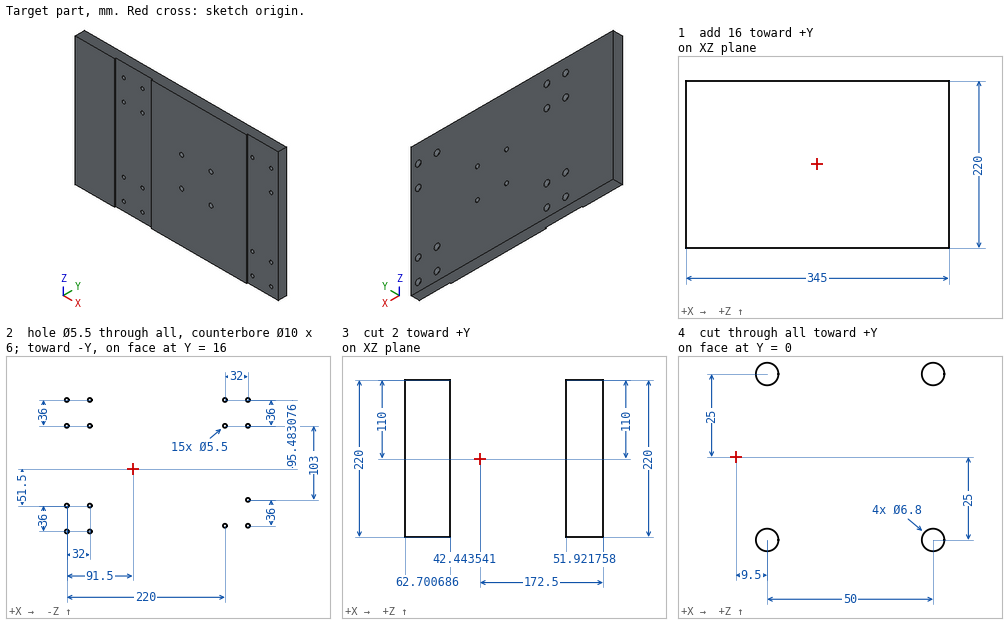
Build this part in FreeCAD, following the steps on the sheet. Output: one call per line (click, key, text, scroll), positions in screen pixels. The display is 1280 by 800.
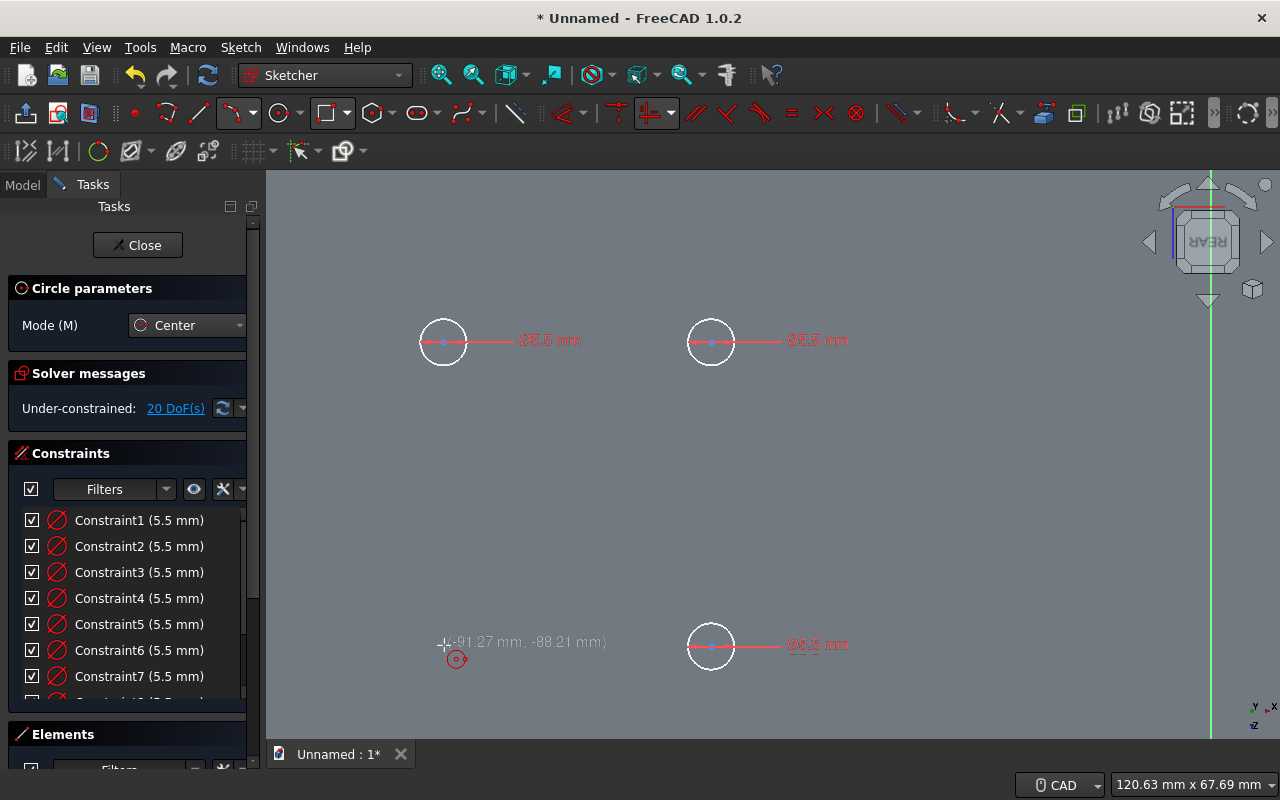
scroll(444, 645, down, 7)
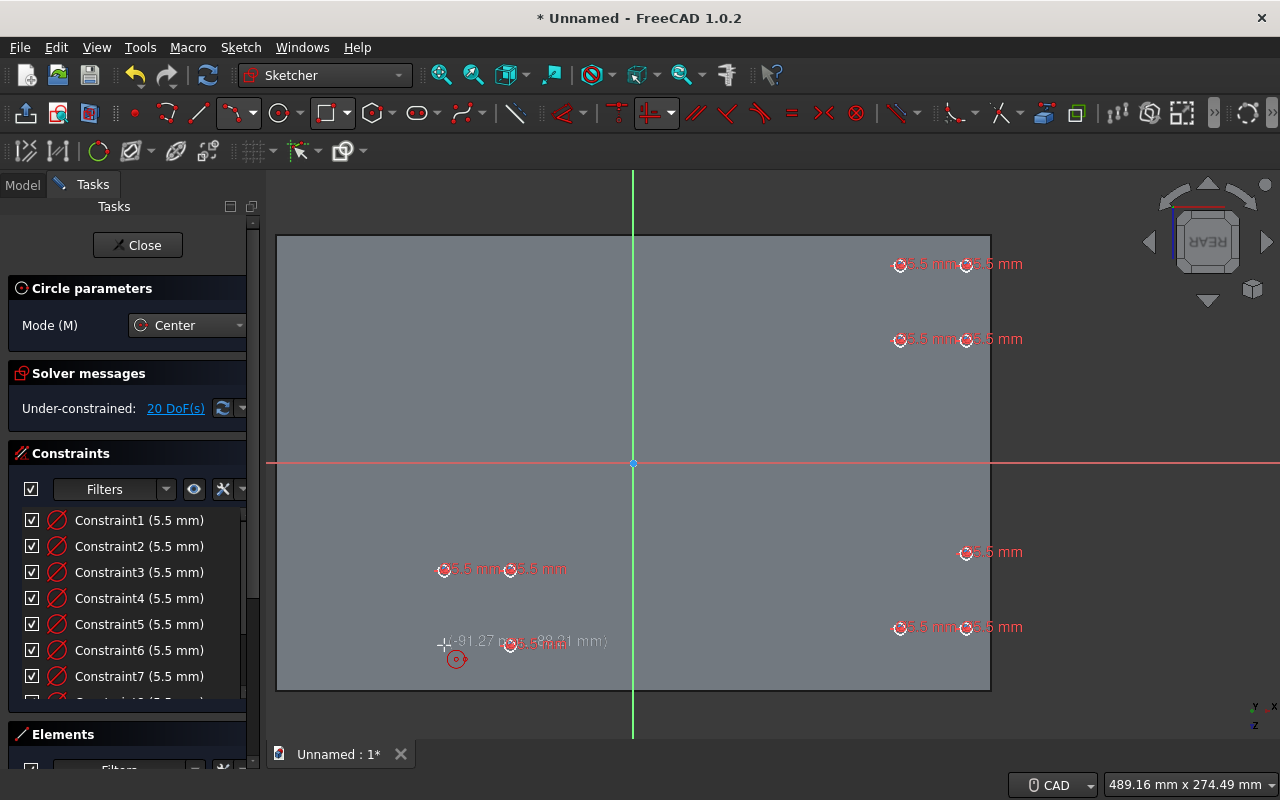
click(444, 645)
move(448, 640)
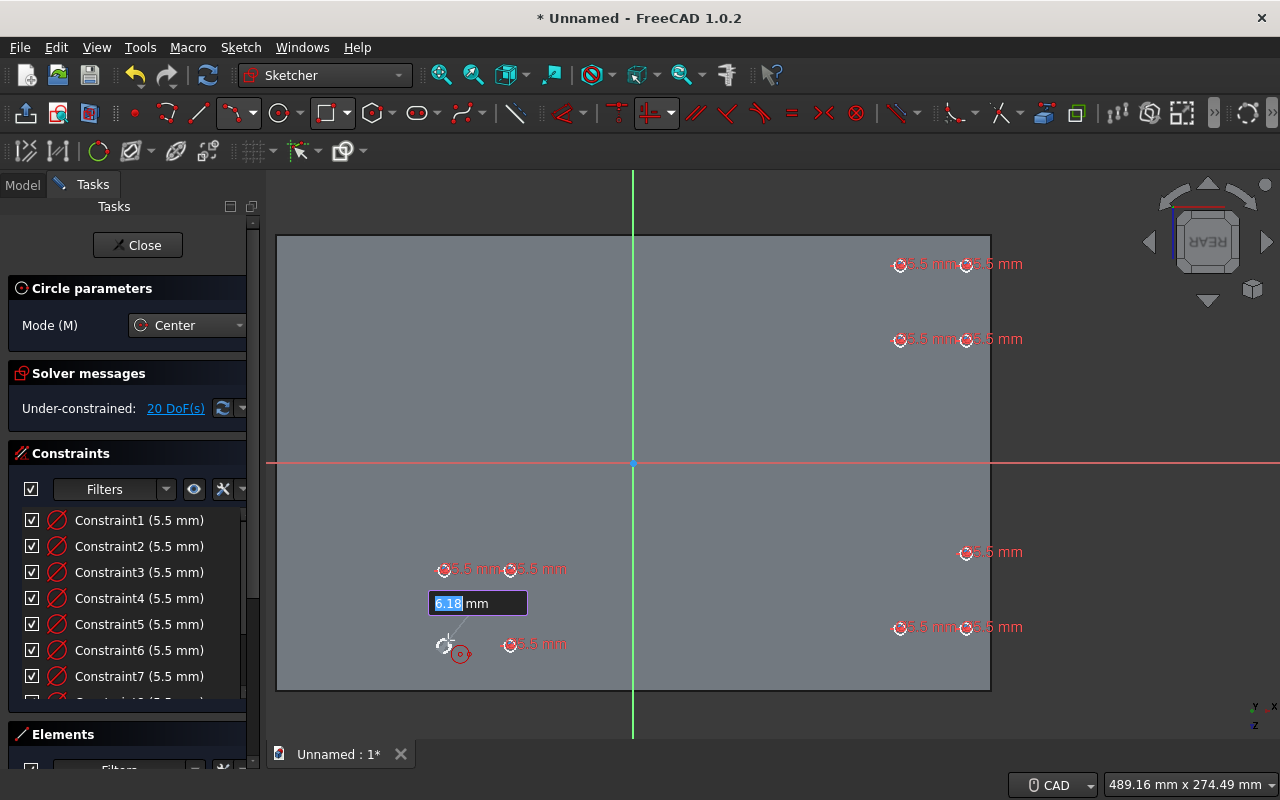
text(5.5)
key(Return)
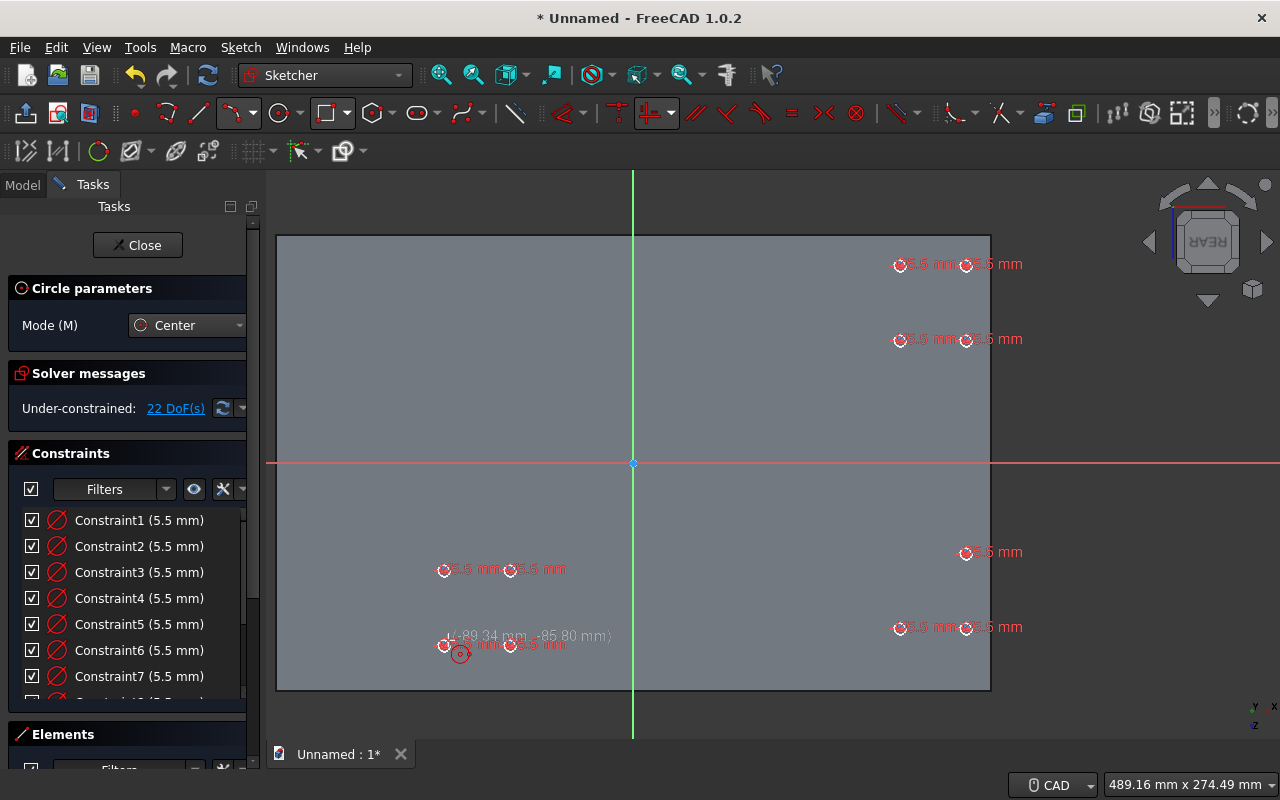
scroll(444, 340, up, 7)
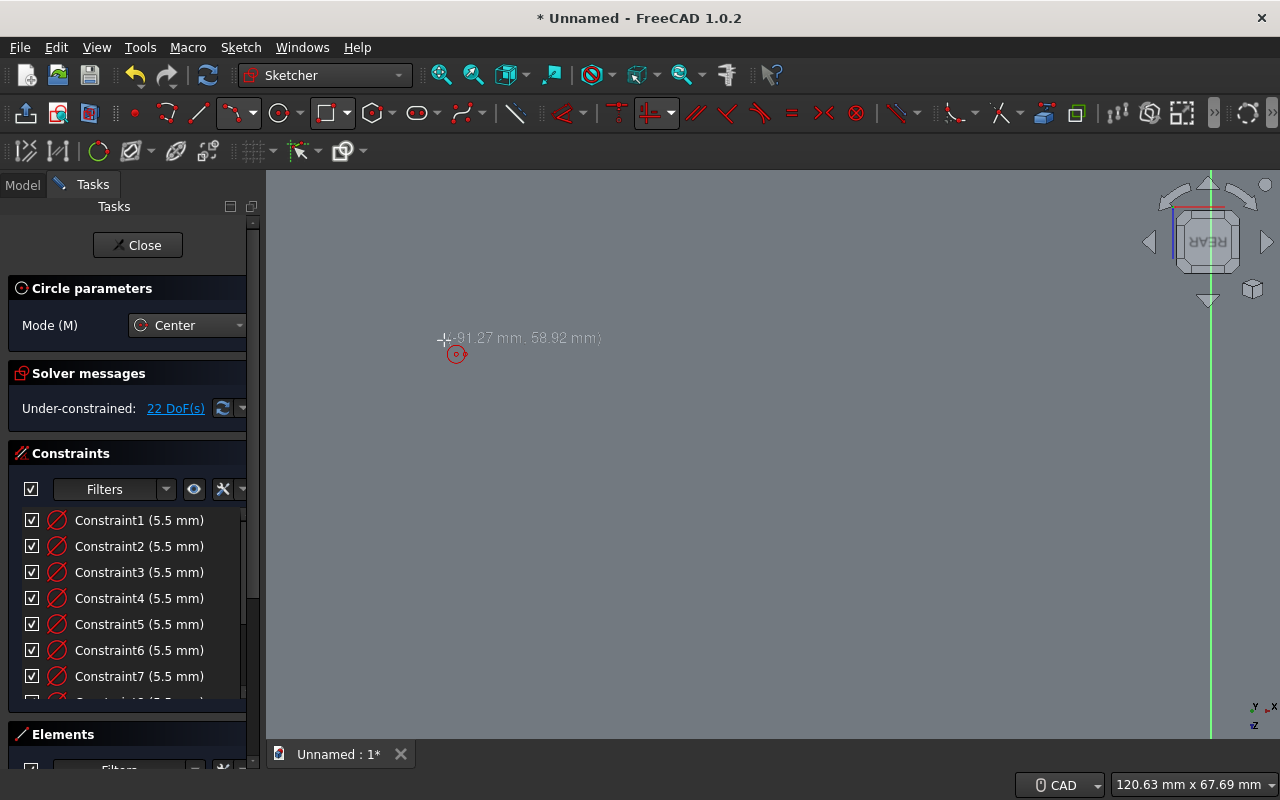
scroll(444, 340, down, 7)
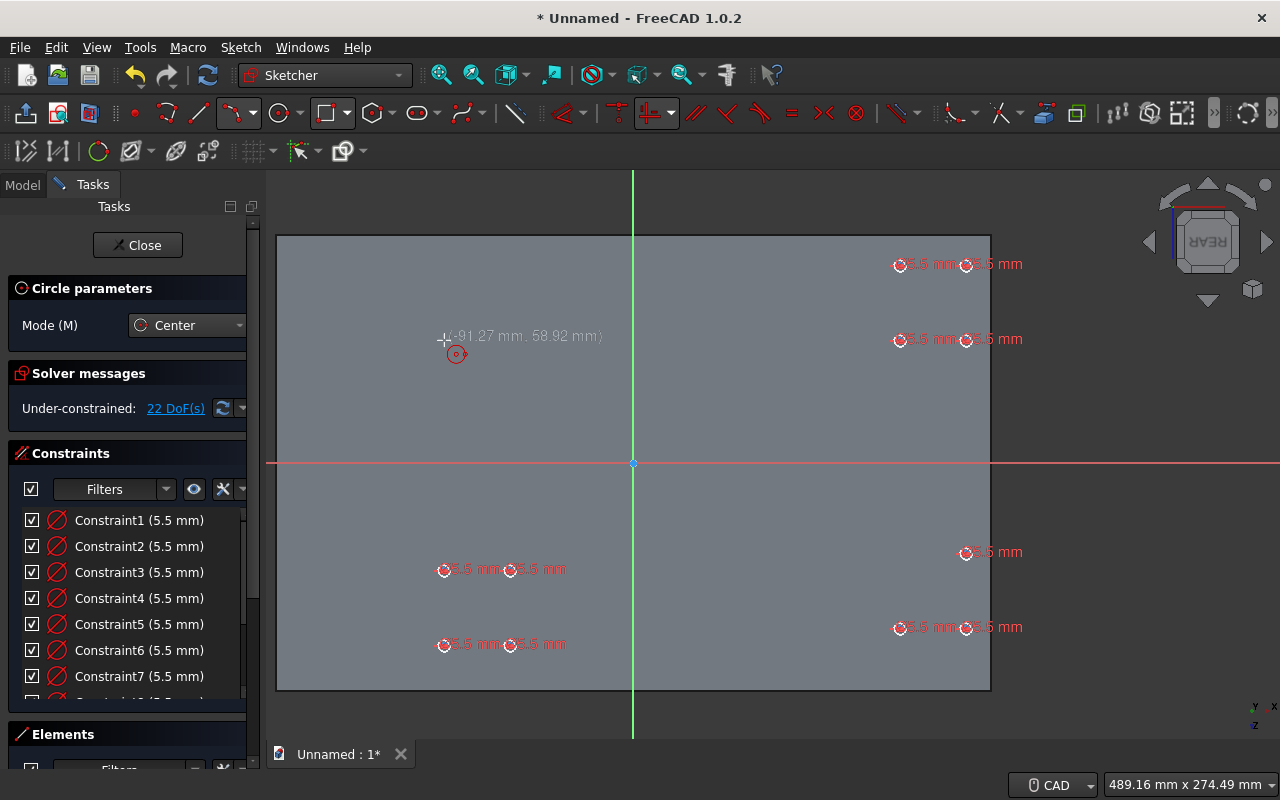
click(444, 340)
move(448, 336)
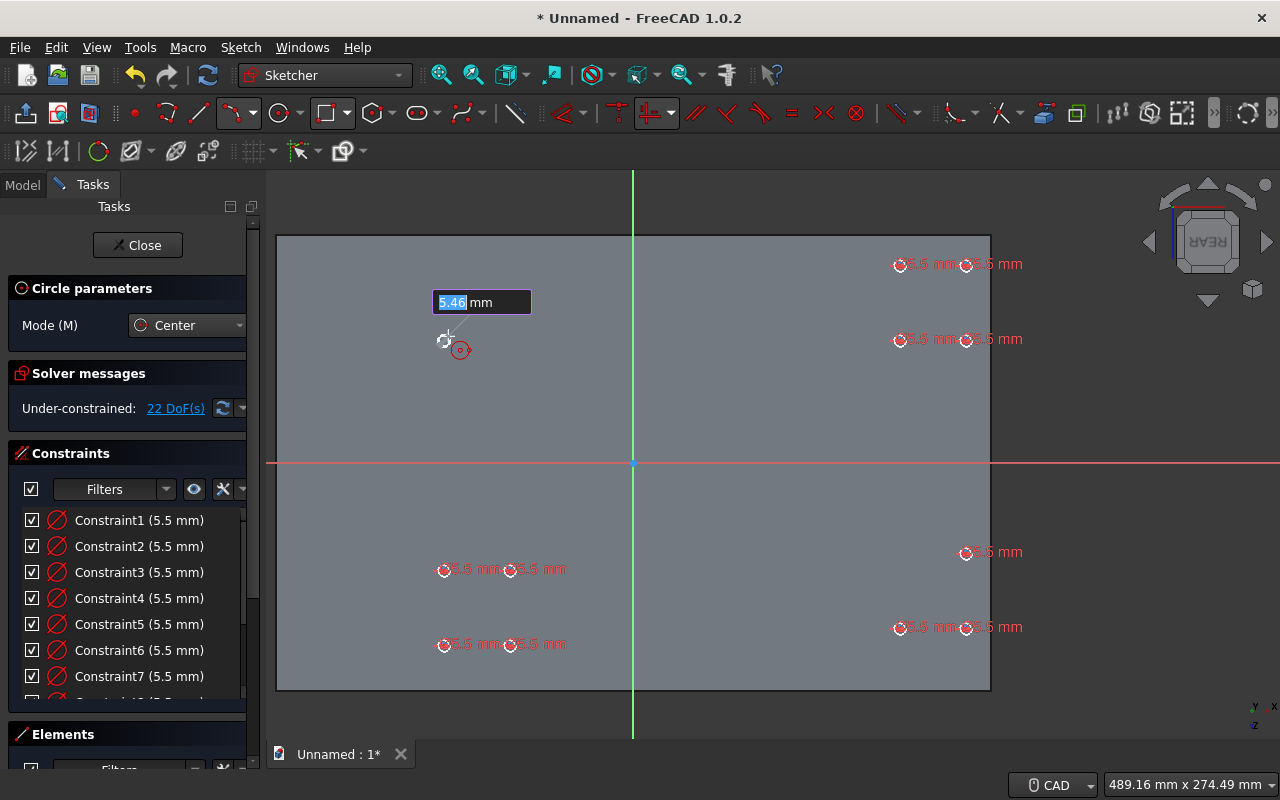
text(5.5)
key(Return)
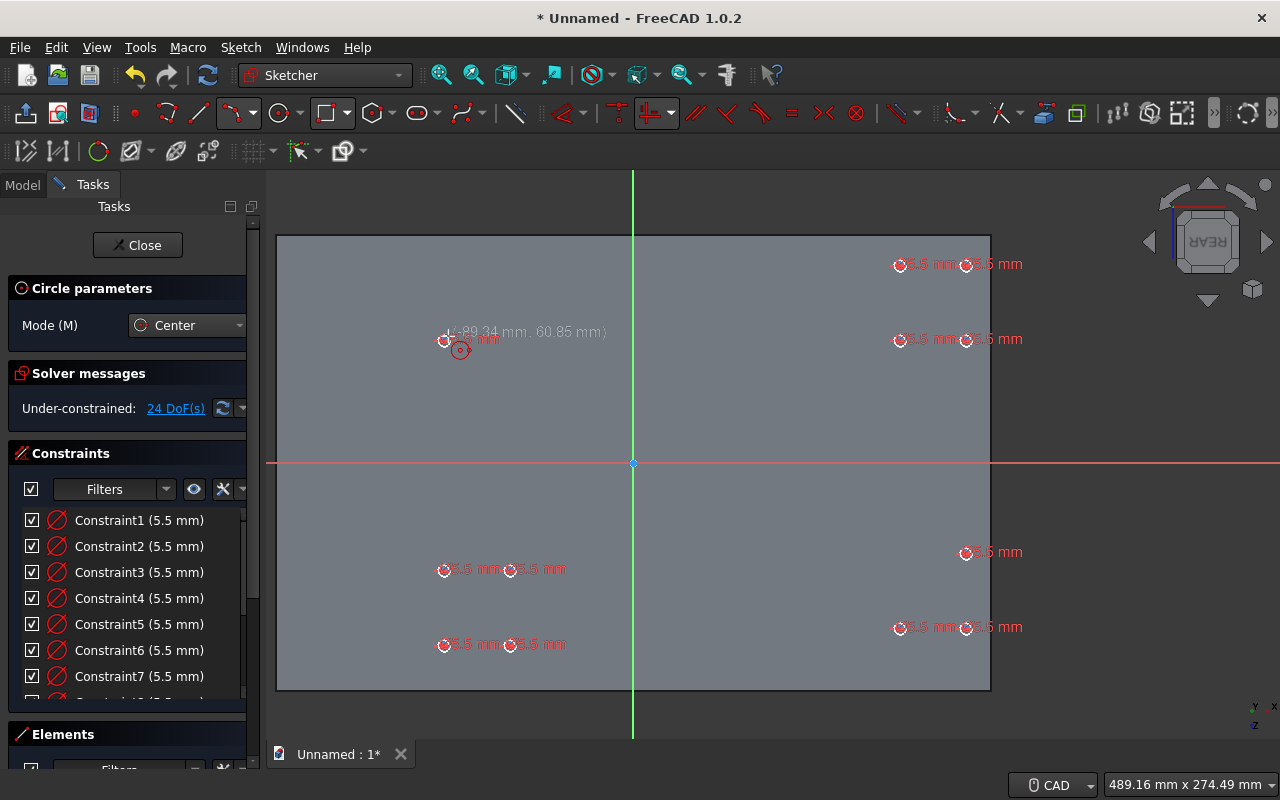
scroll(510, 340, up, 7)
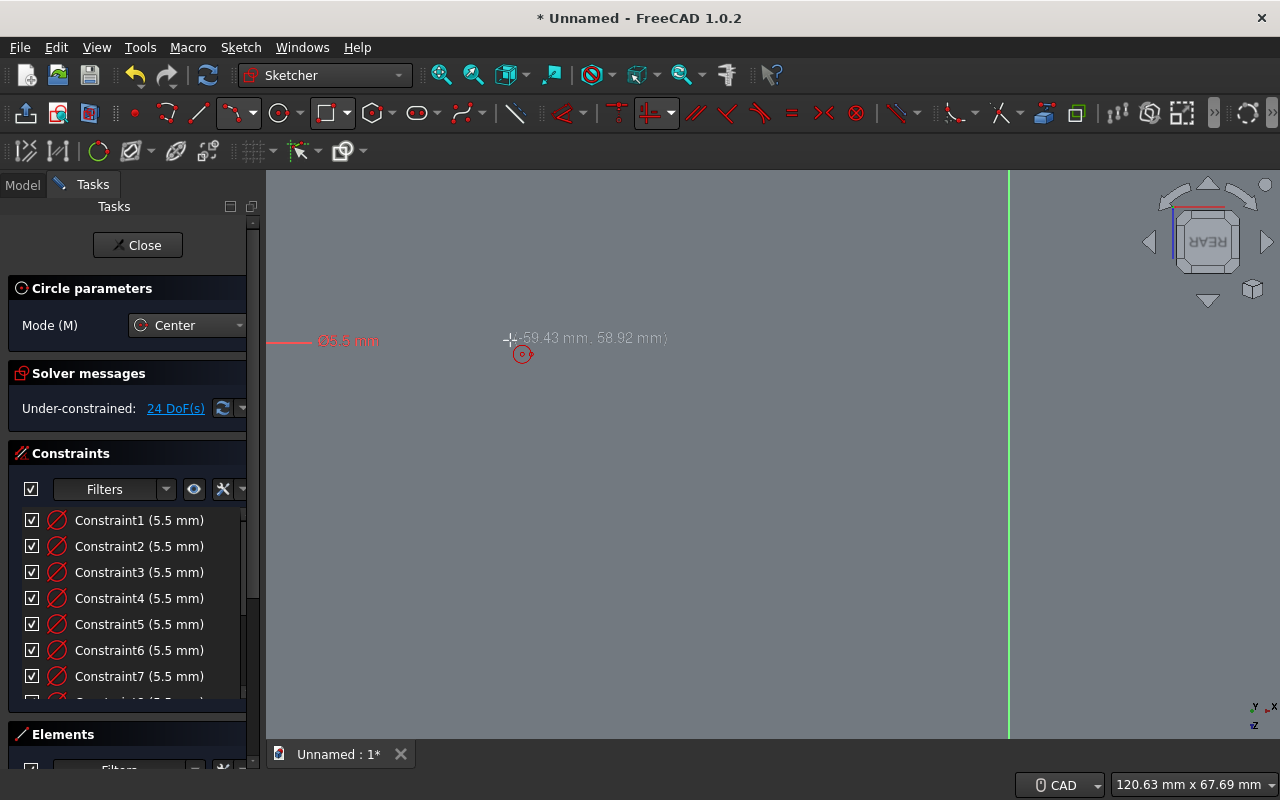
scroll(510, 340, down, 7)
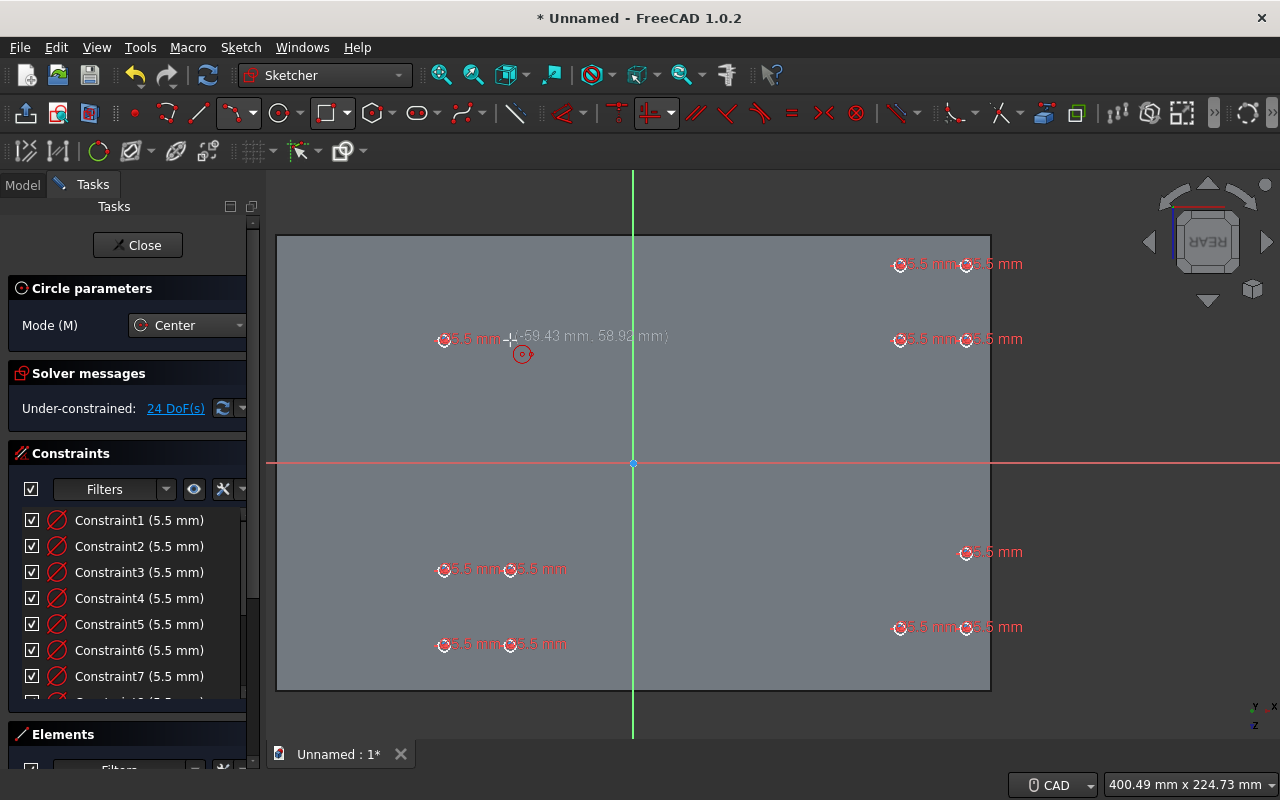
click(510, 340)
move(514, 336)